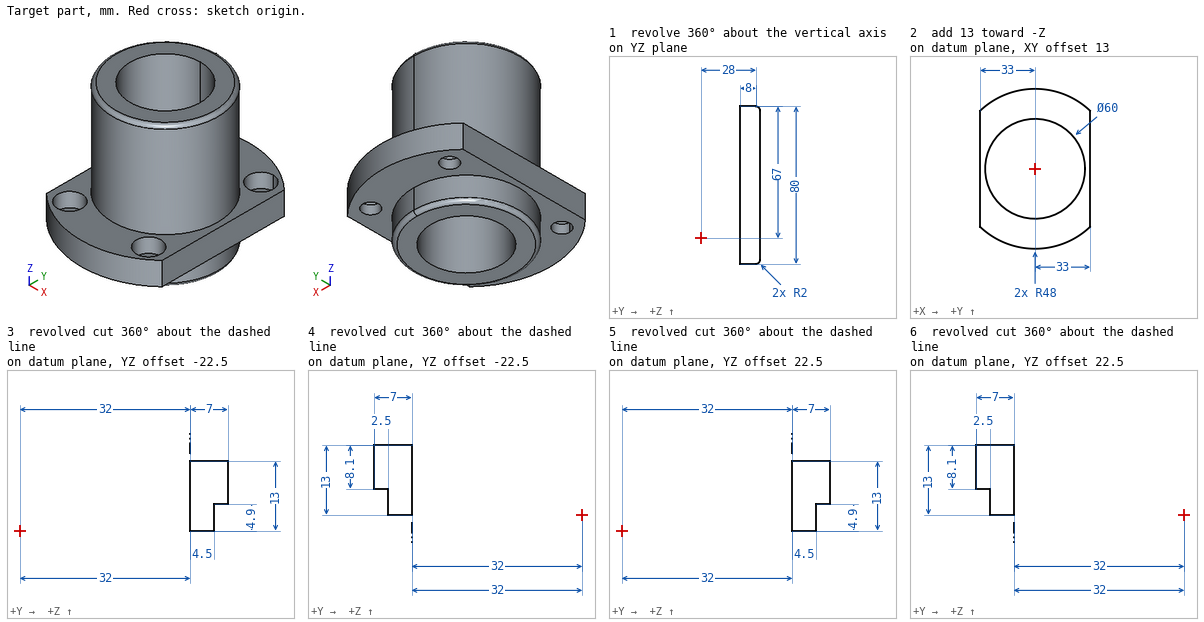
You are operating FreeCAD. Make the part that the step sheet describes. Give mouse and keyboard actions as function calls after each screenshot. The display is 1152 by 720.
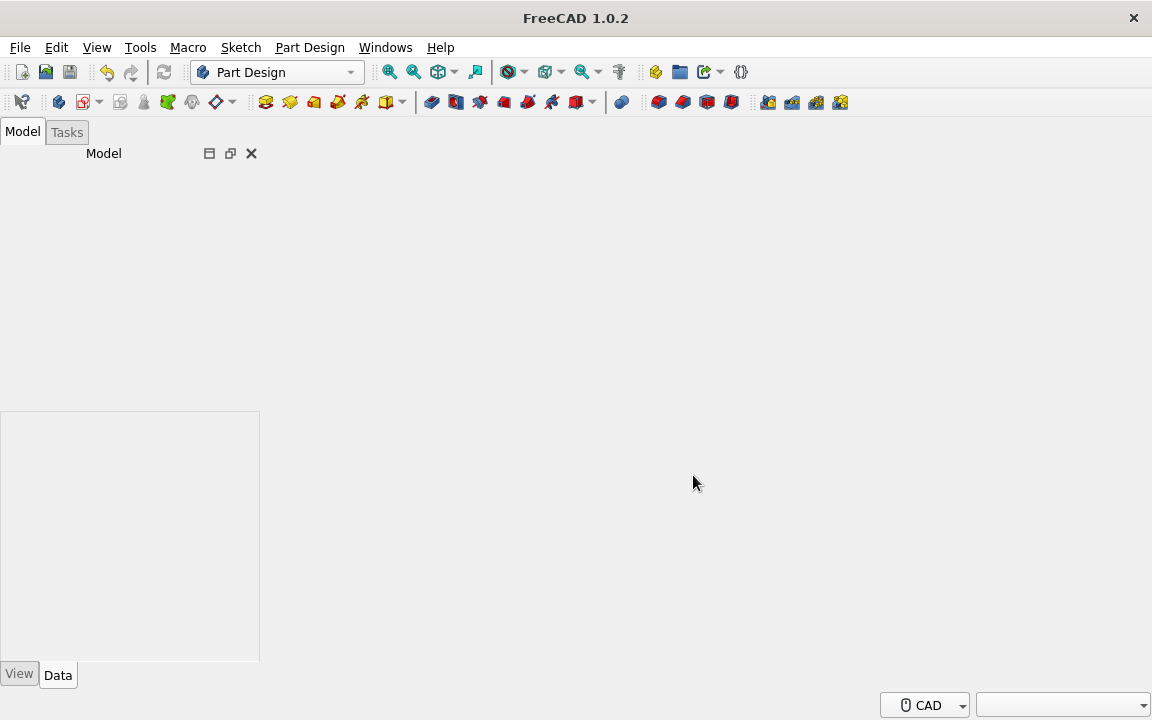
click(22, 72)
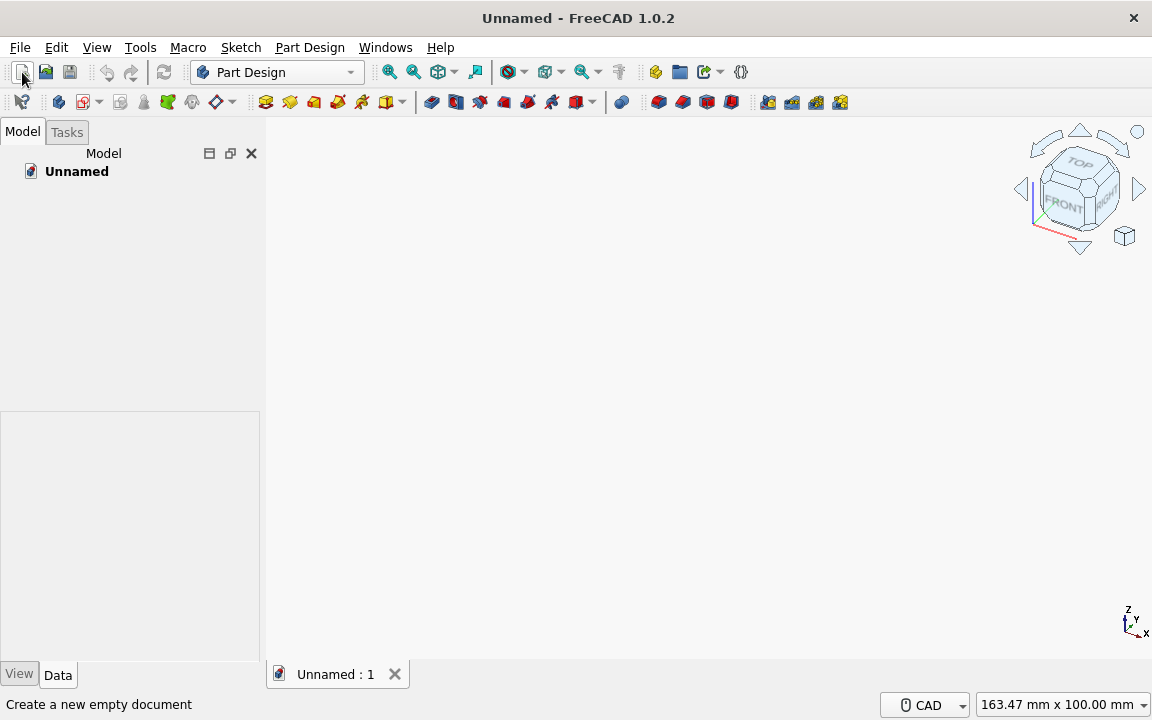
click(84, 102)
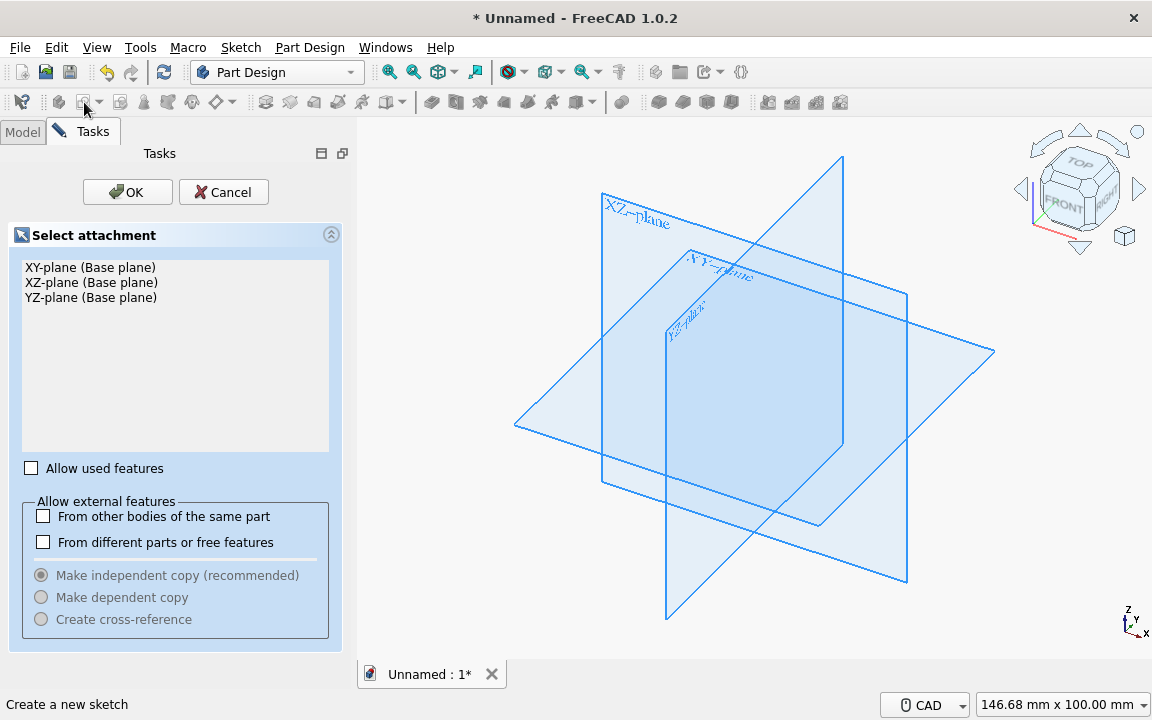
click(82, 298)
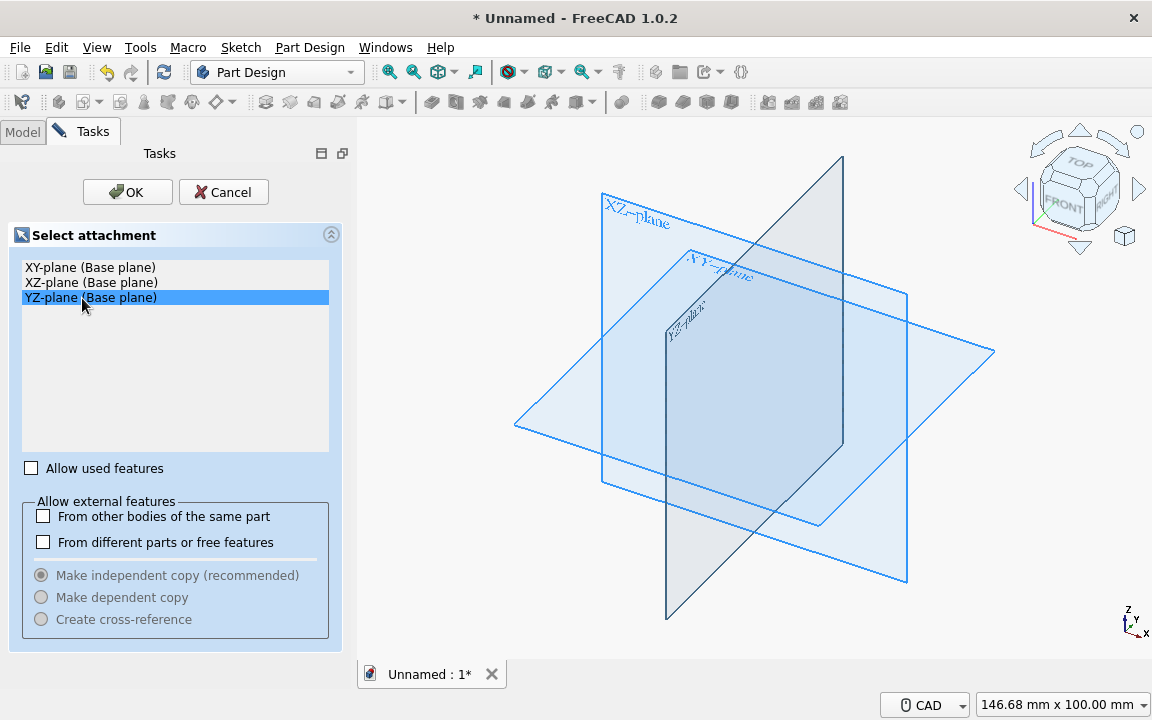
click(128, 192)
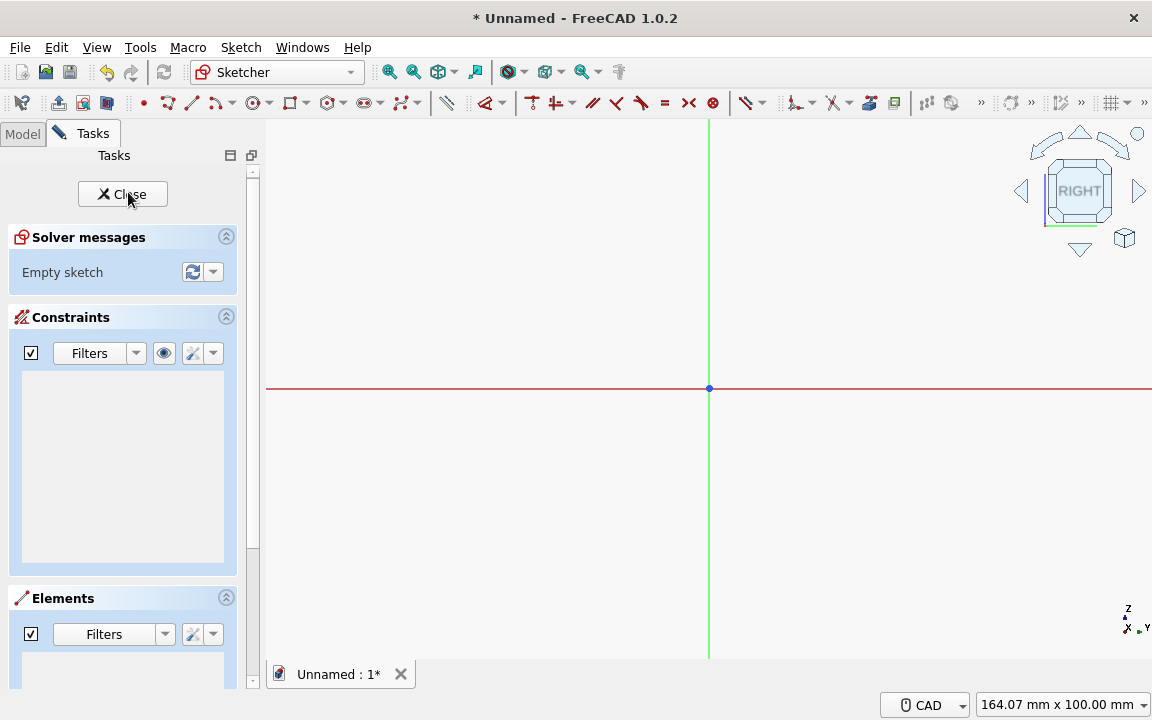
scroll(337, 631, down, 2)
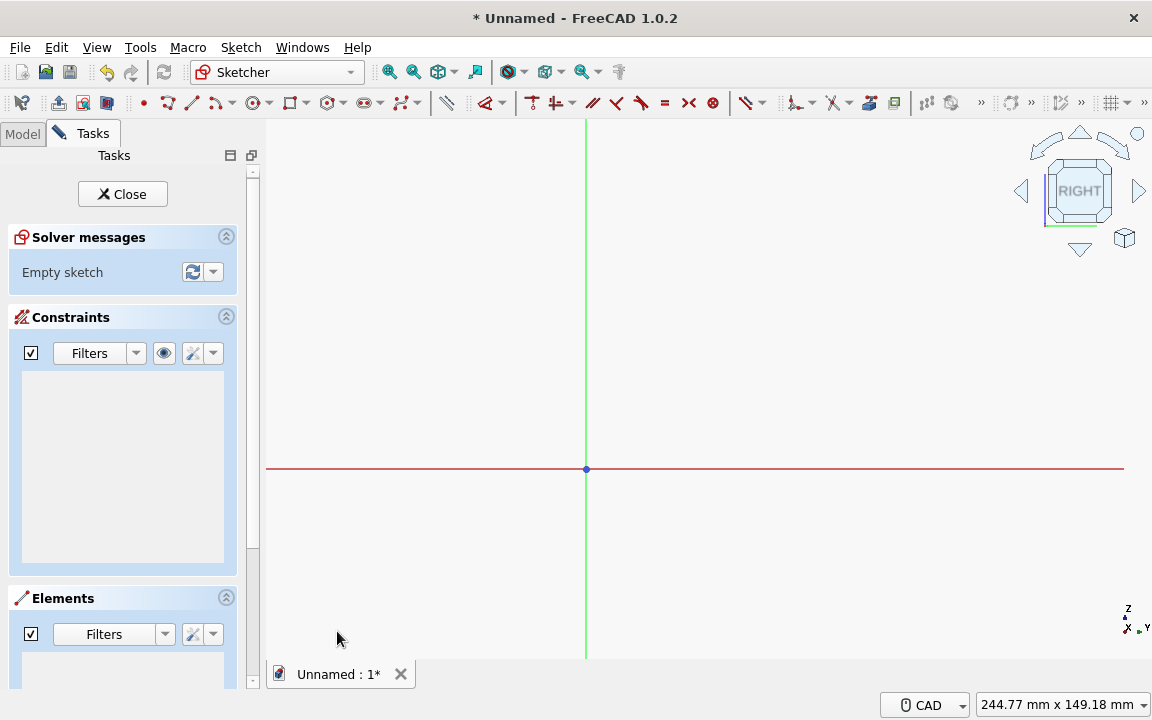
click(168, 104)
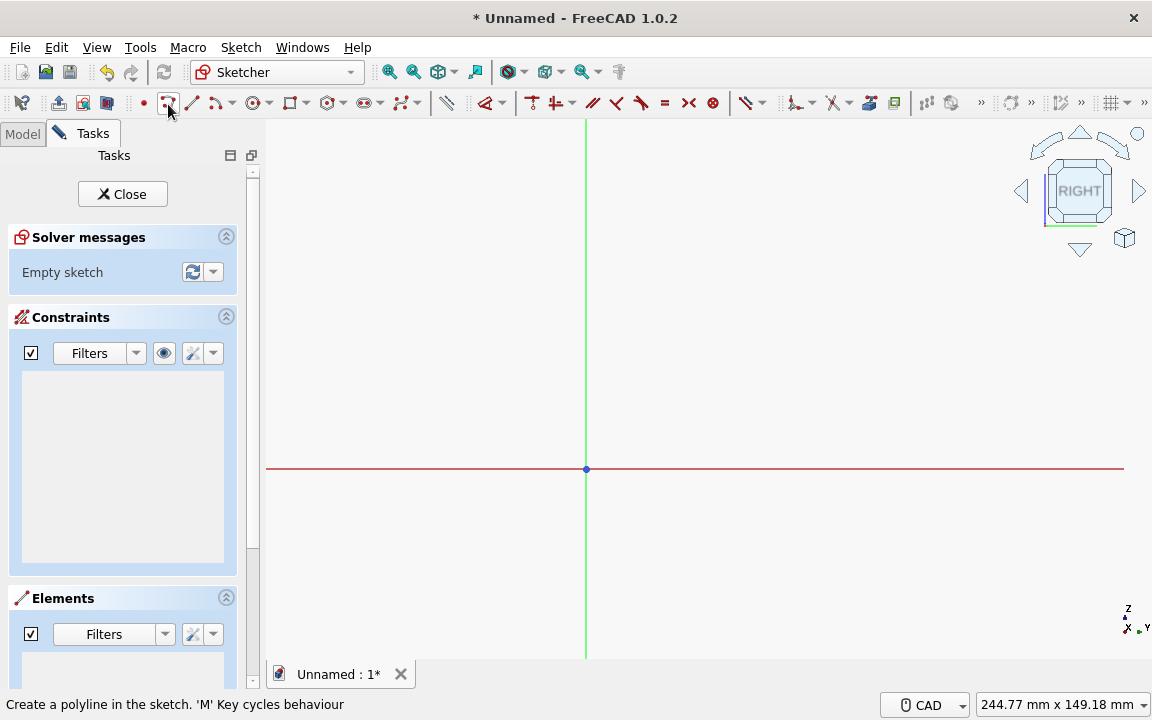
click(688, 227)
click(659, 227)
click(659, 516)
click(688, 516)
right_click(688, 516)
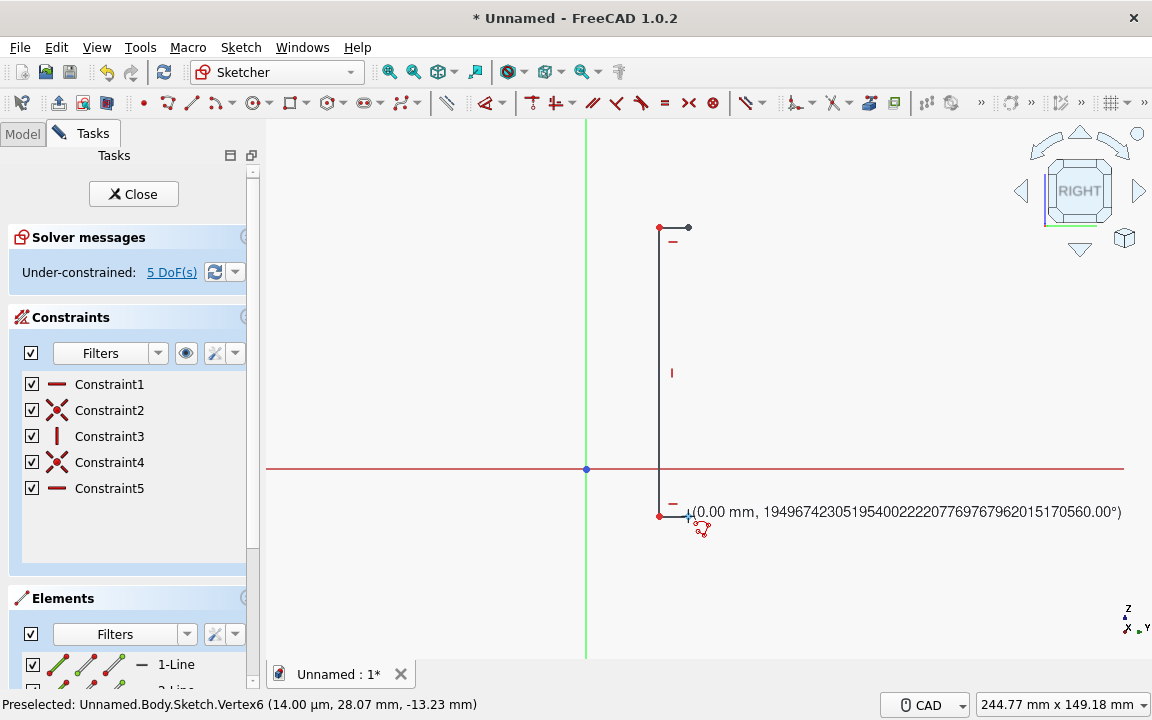
click(192, 104)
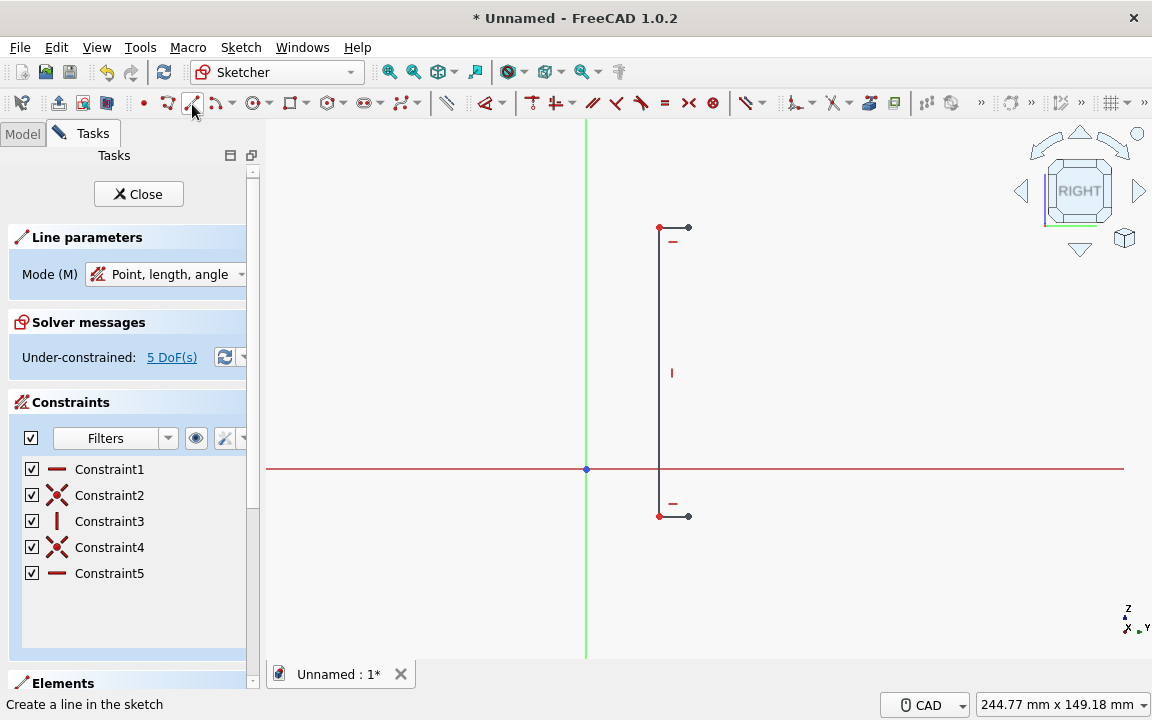
scroll(695, 509, up, 3)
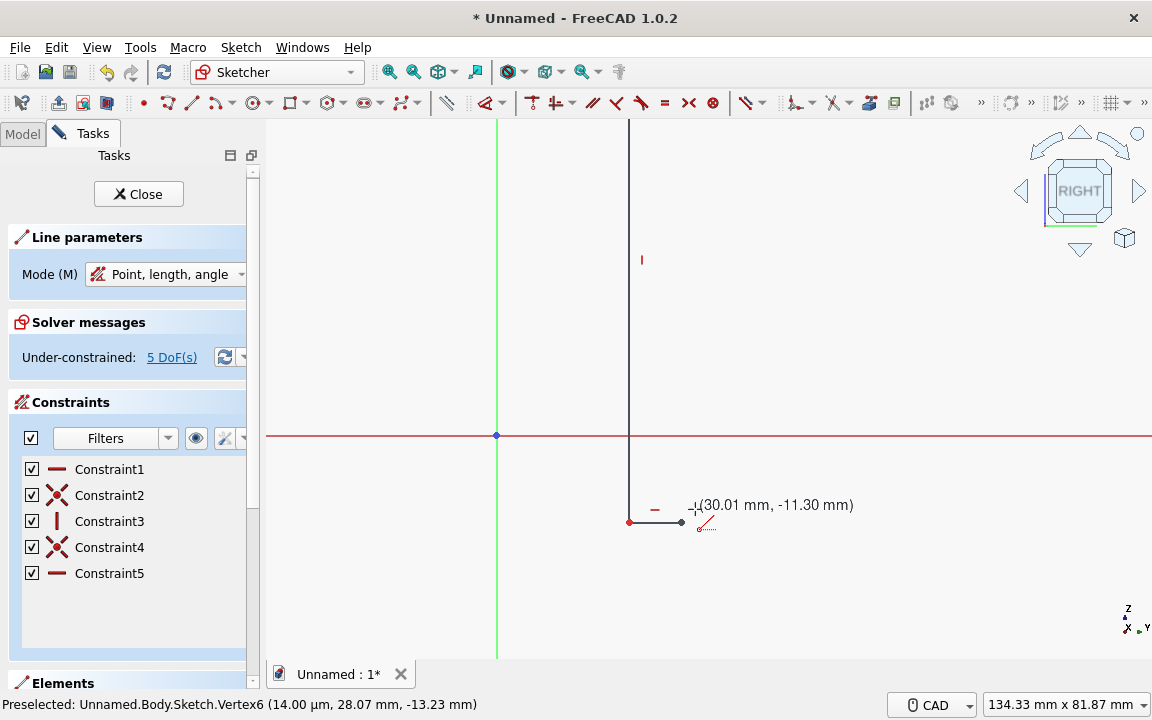
click(695, 508)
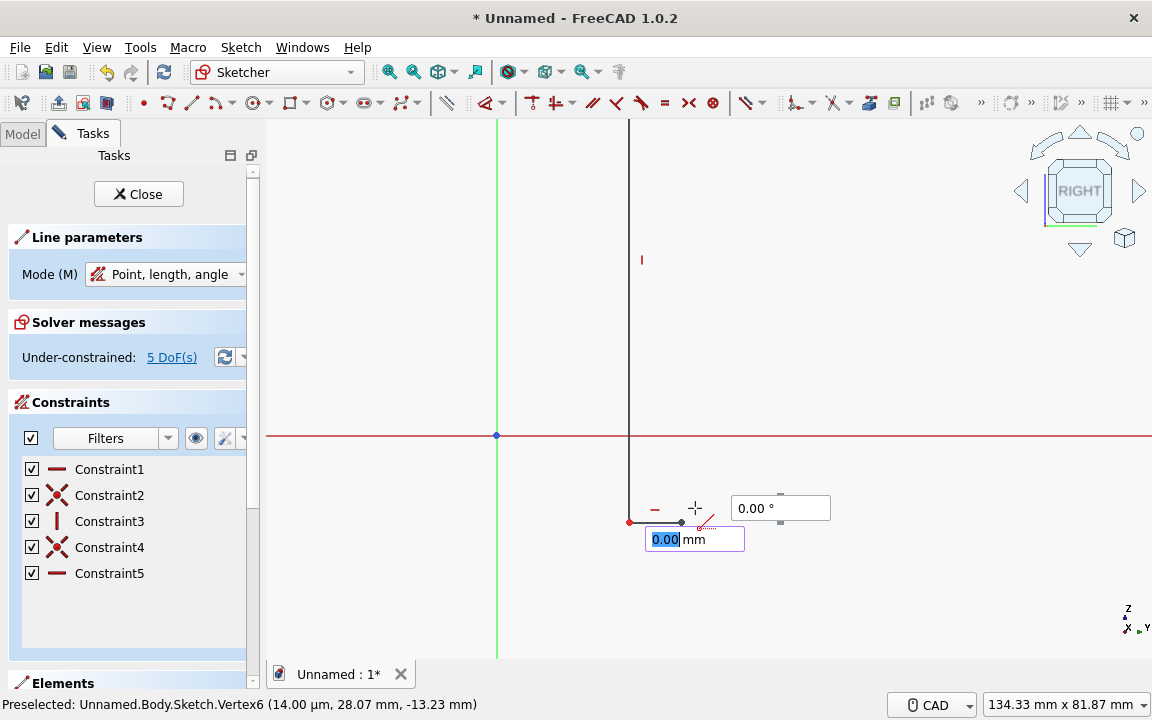
scroll(732, 631, down, 2)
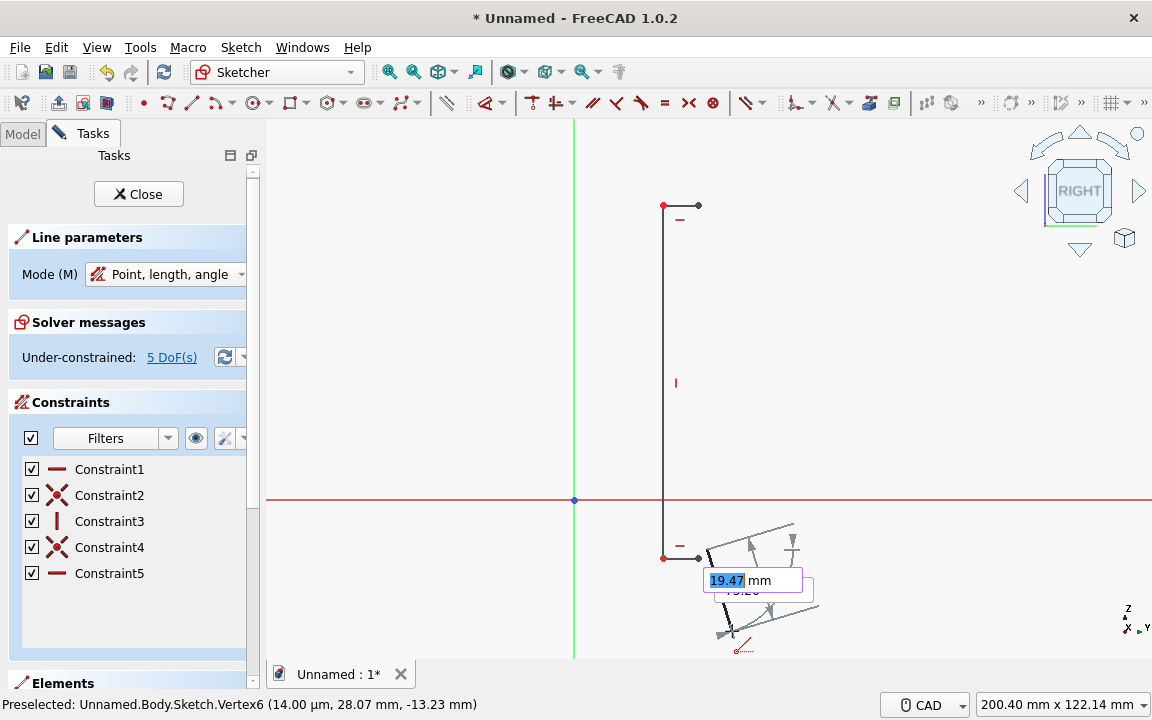
scroll(707, 213, up, 2)